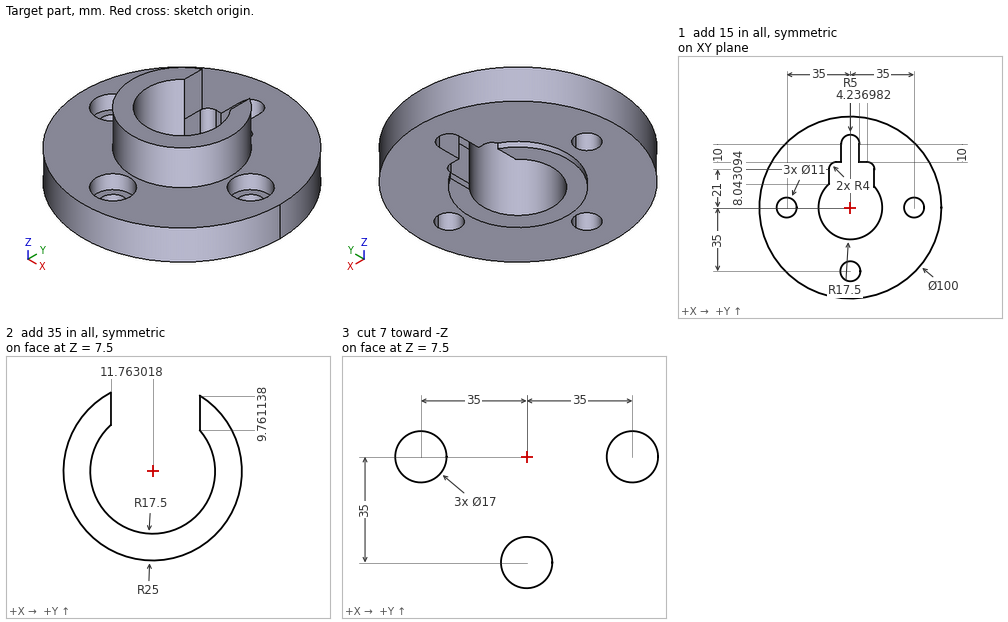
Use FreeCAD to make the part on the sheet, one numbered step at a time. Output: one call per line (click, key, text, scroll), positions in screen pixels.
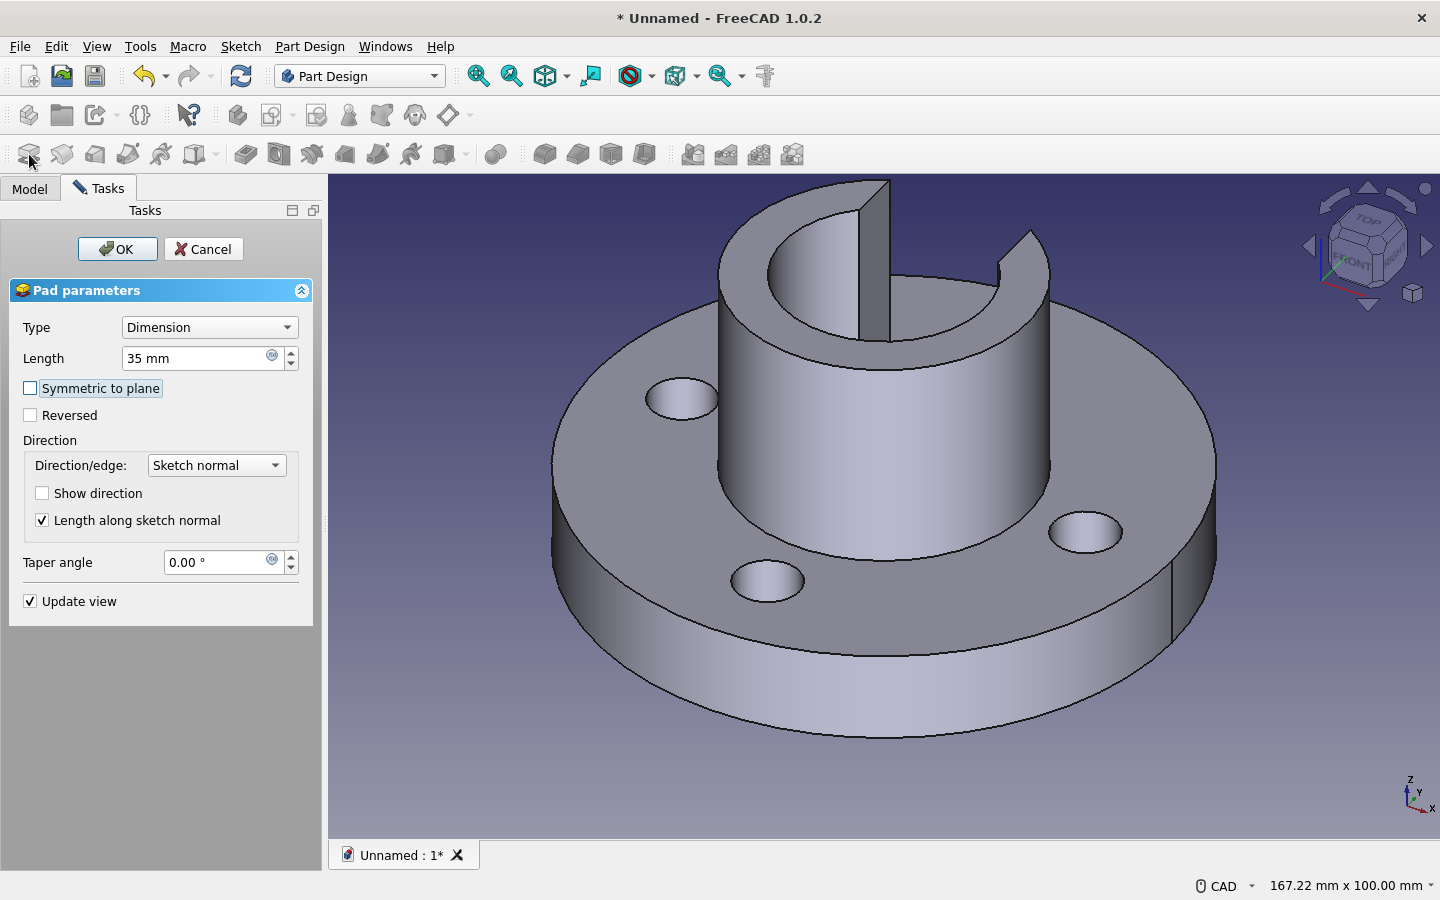
click(31, 388)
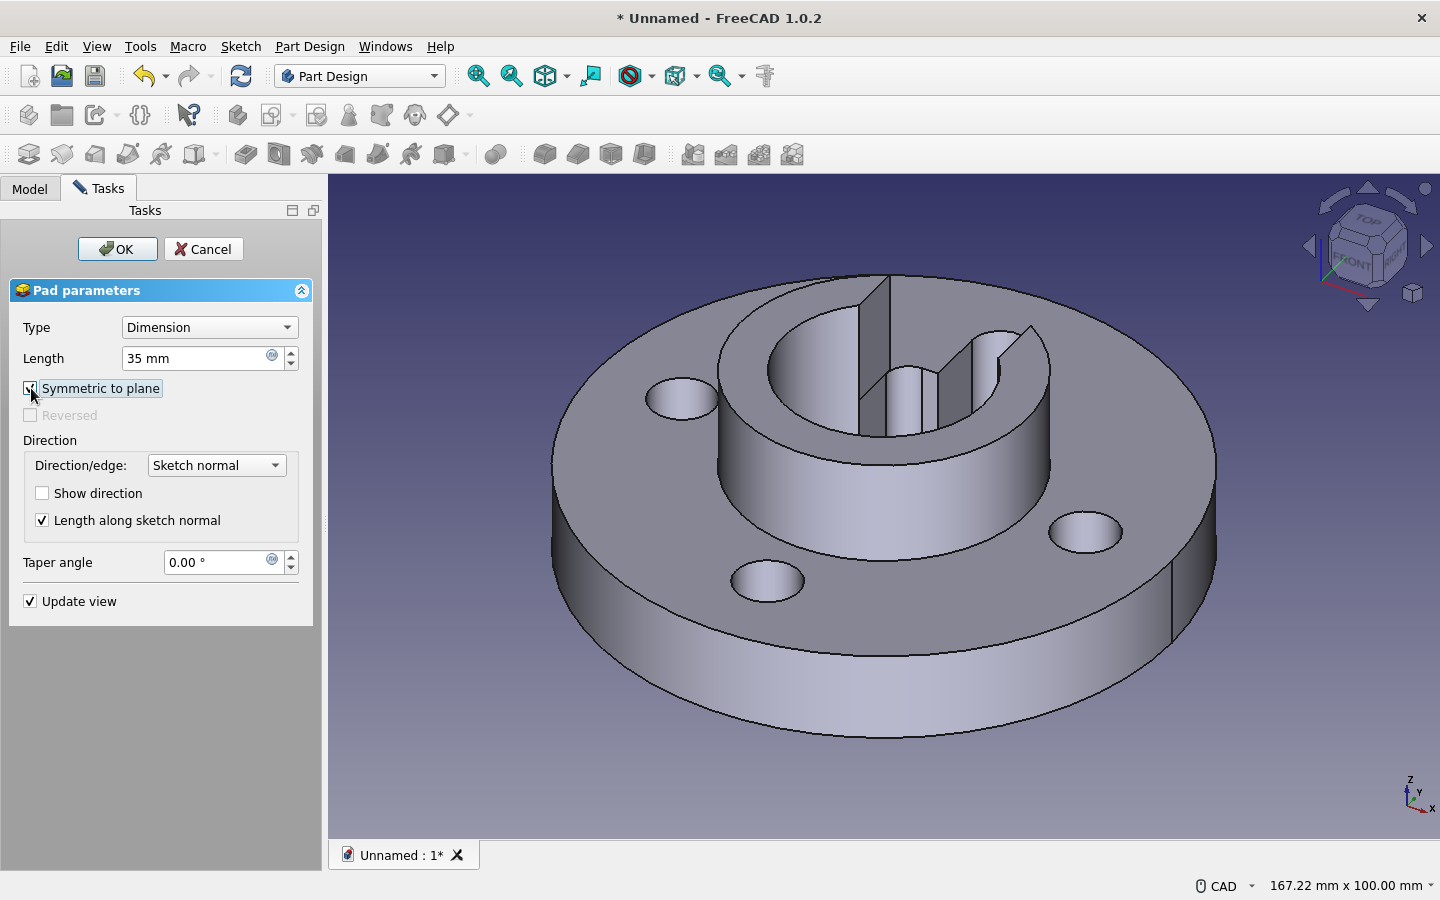
click(118, 249)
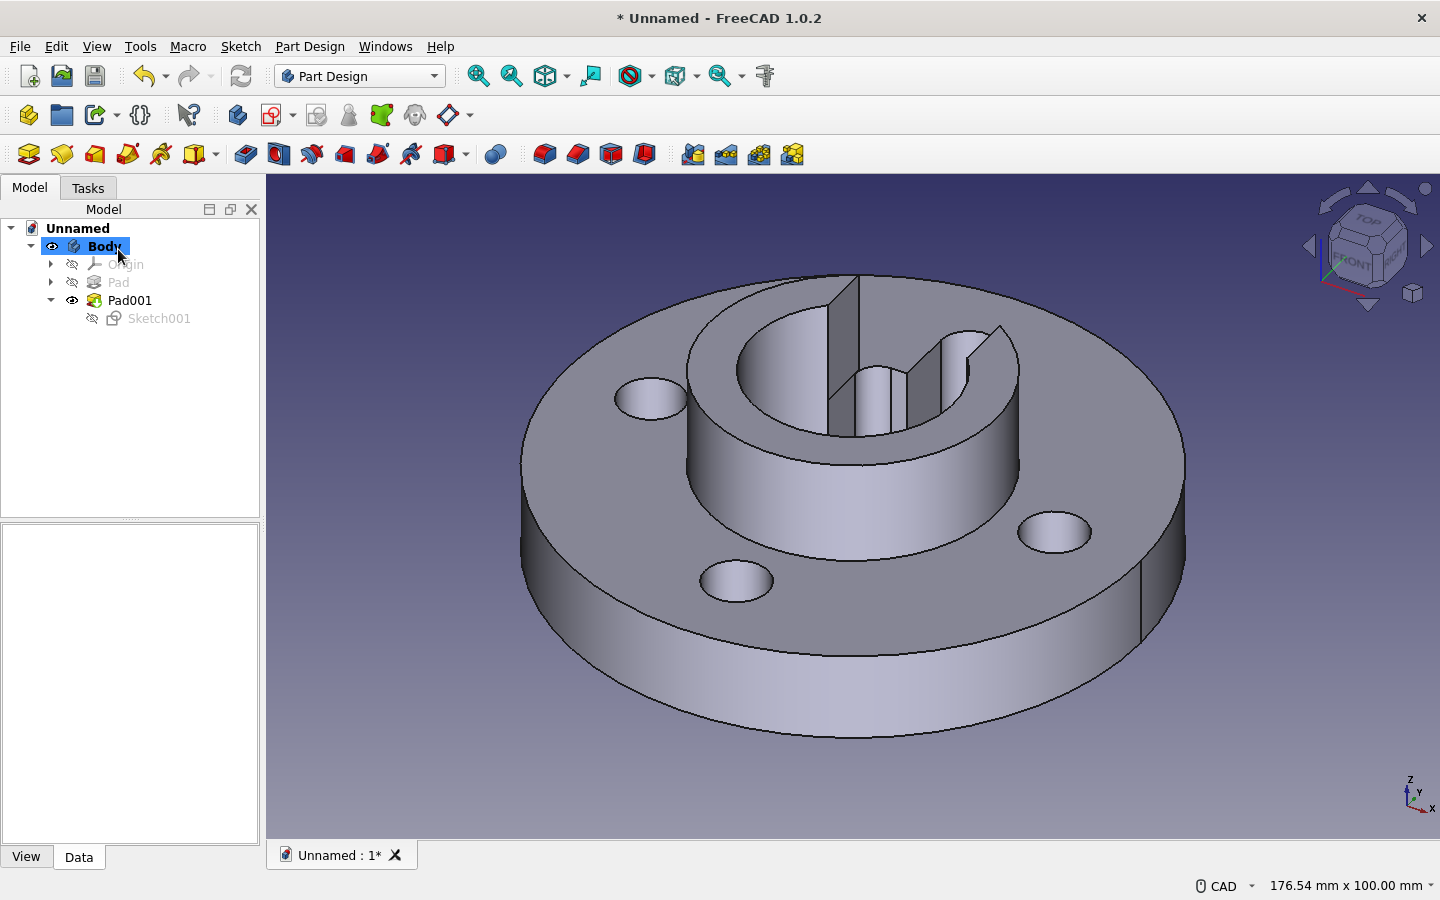
key(v)
key(f)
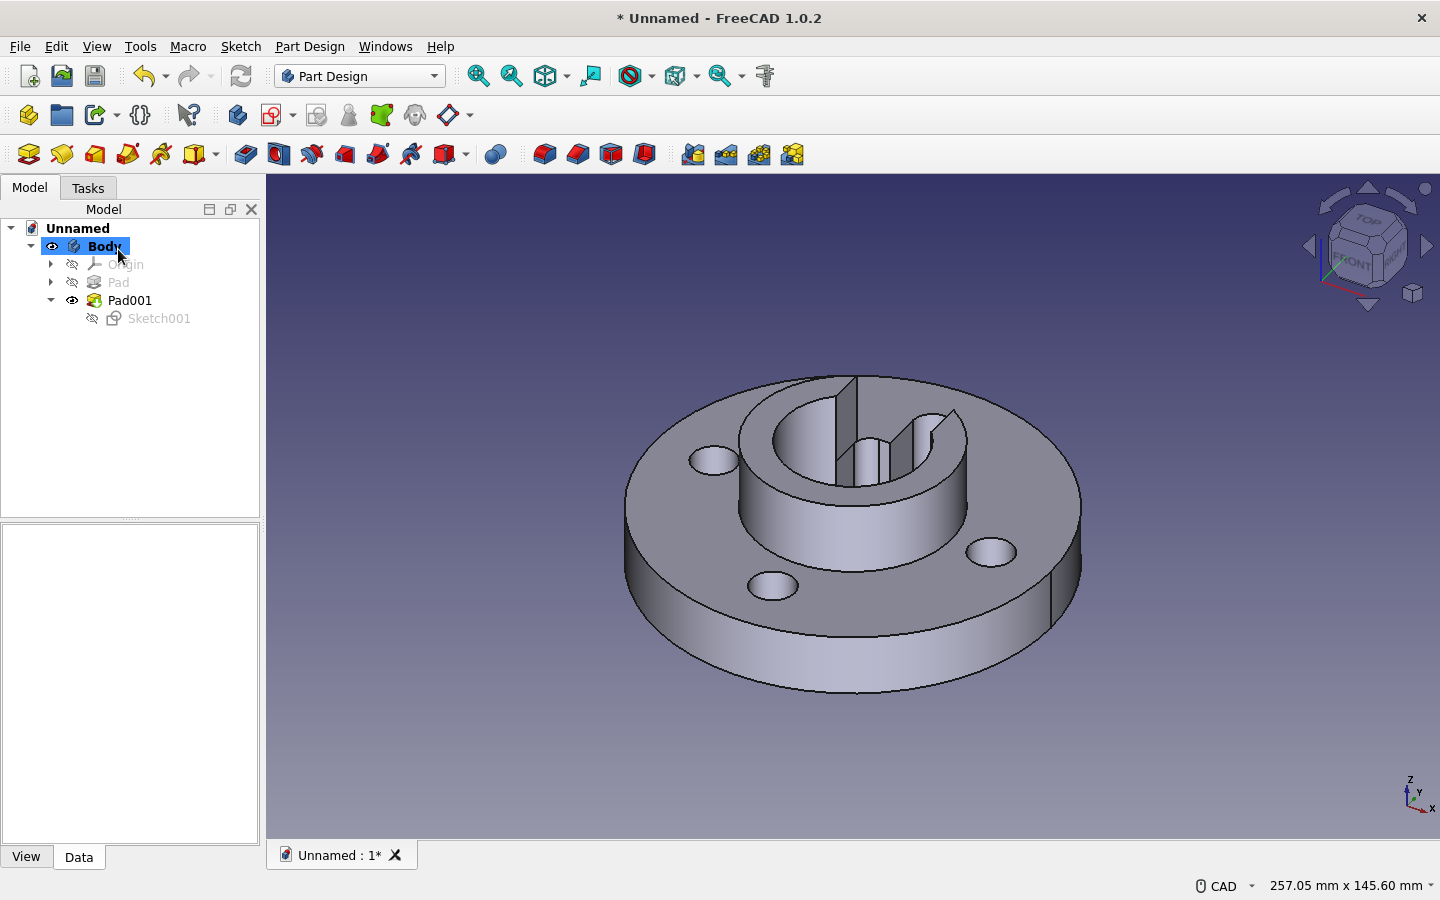
click(901, 608)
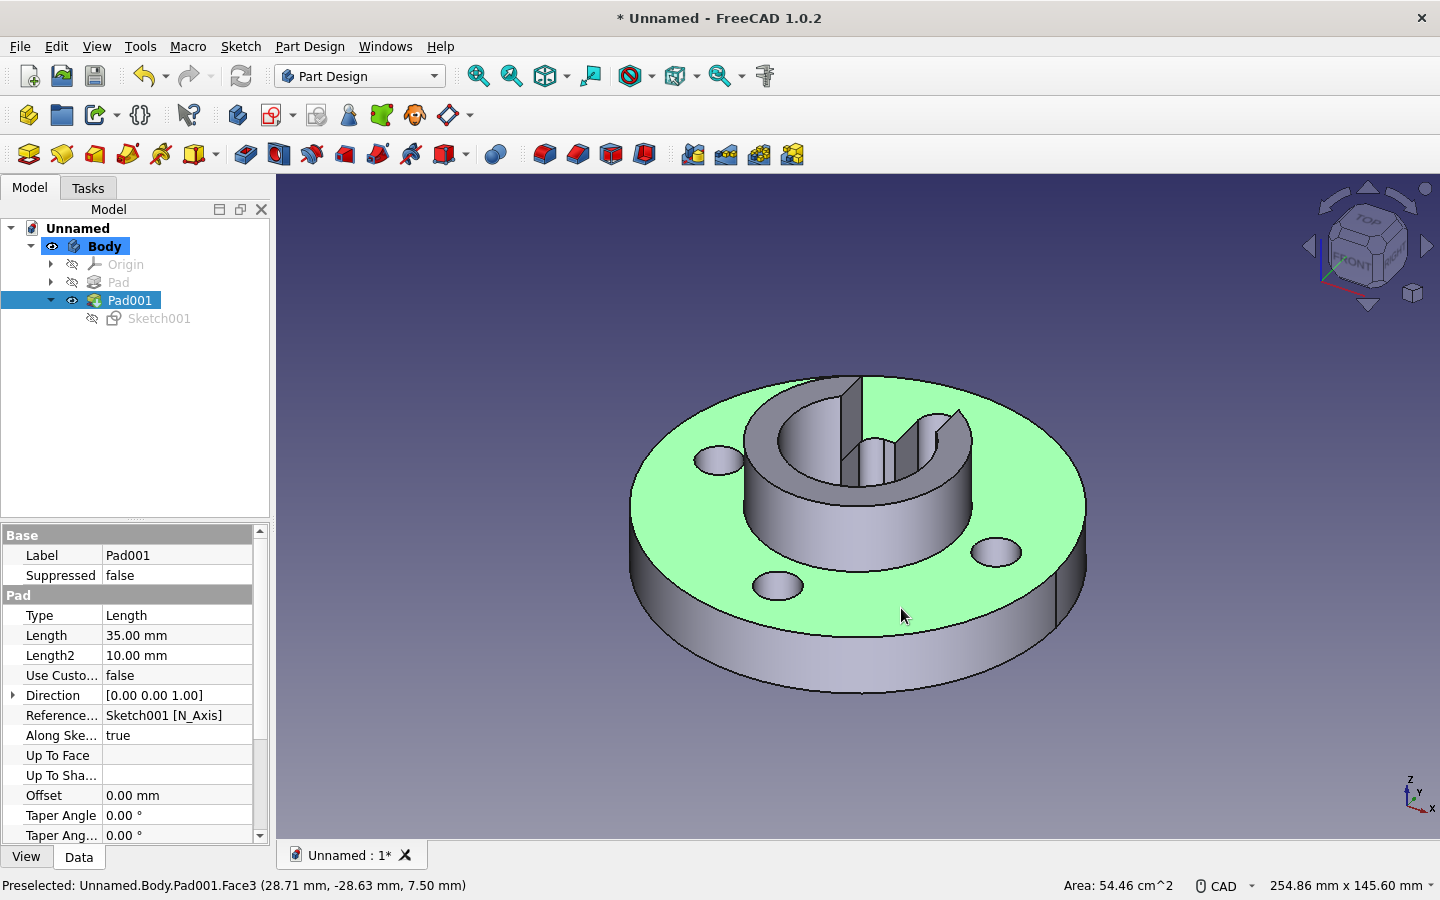
click(270, 116)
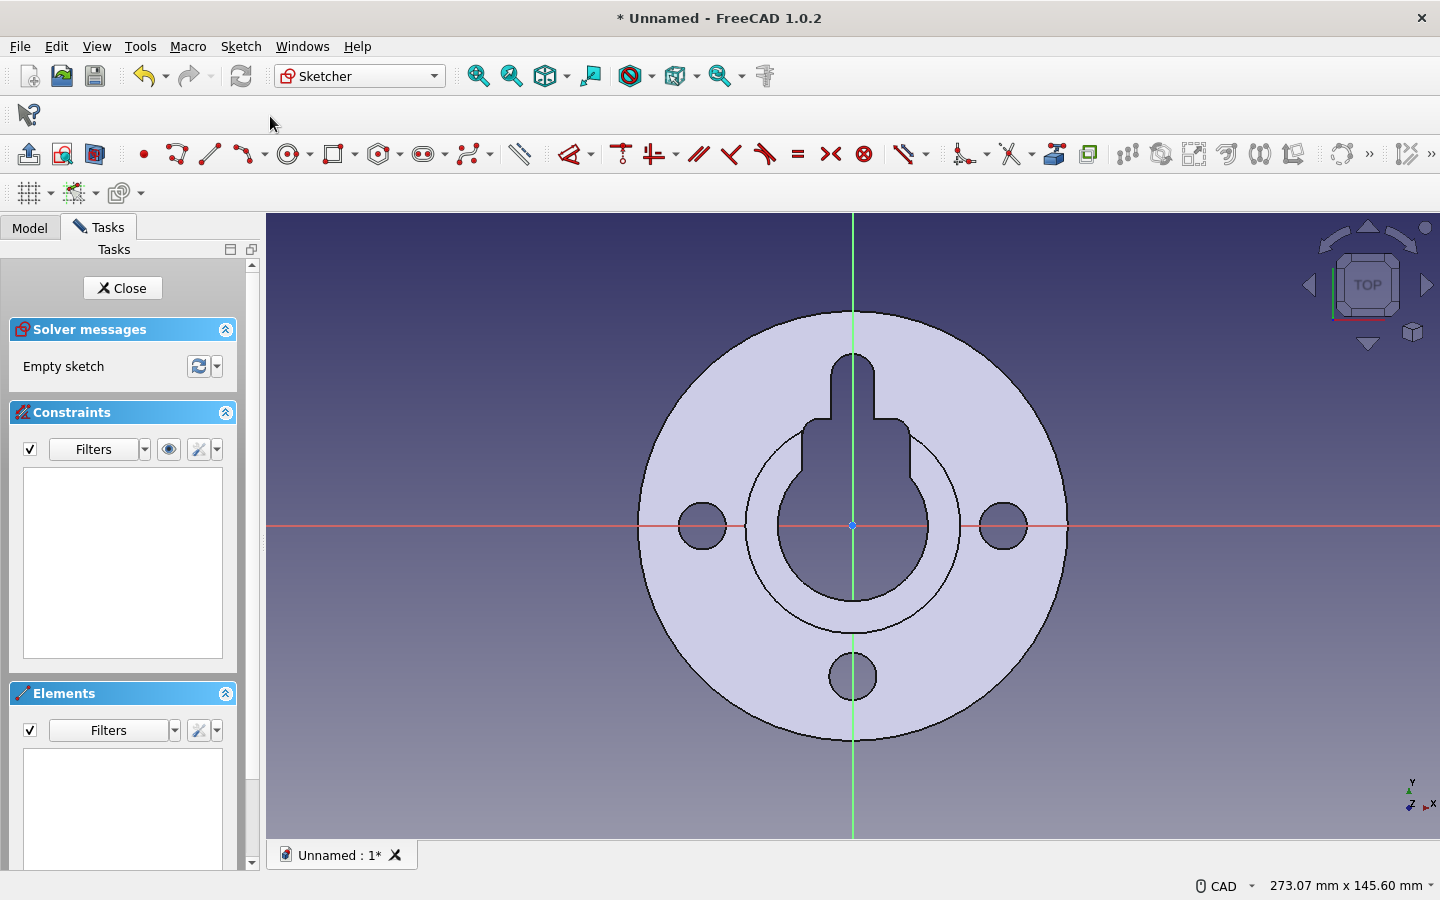
scroll(936, 693, up, 3)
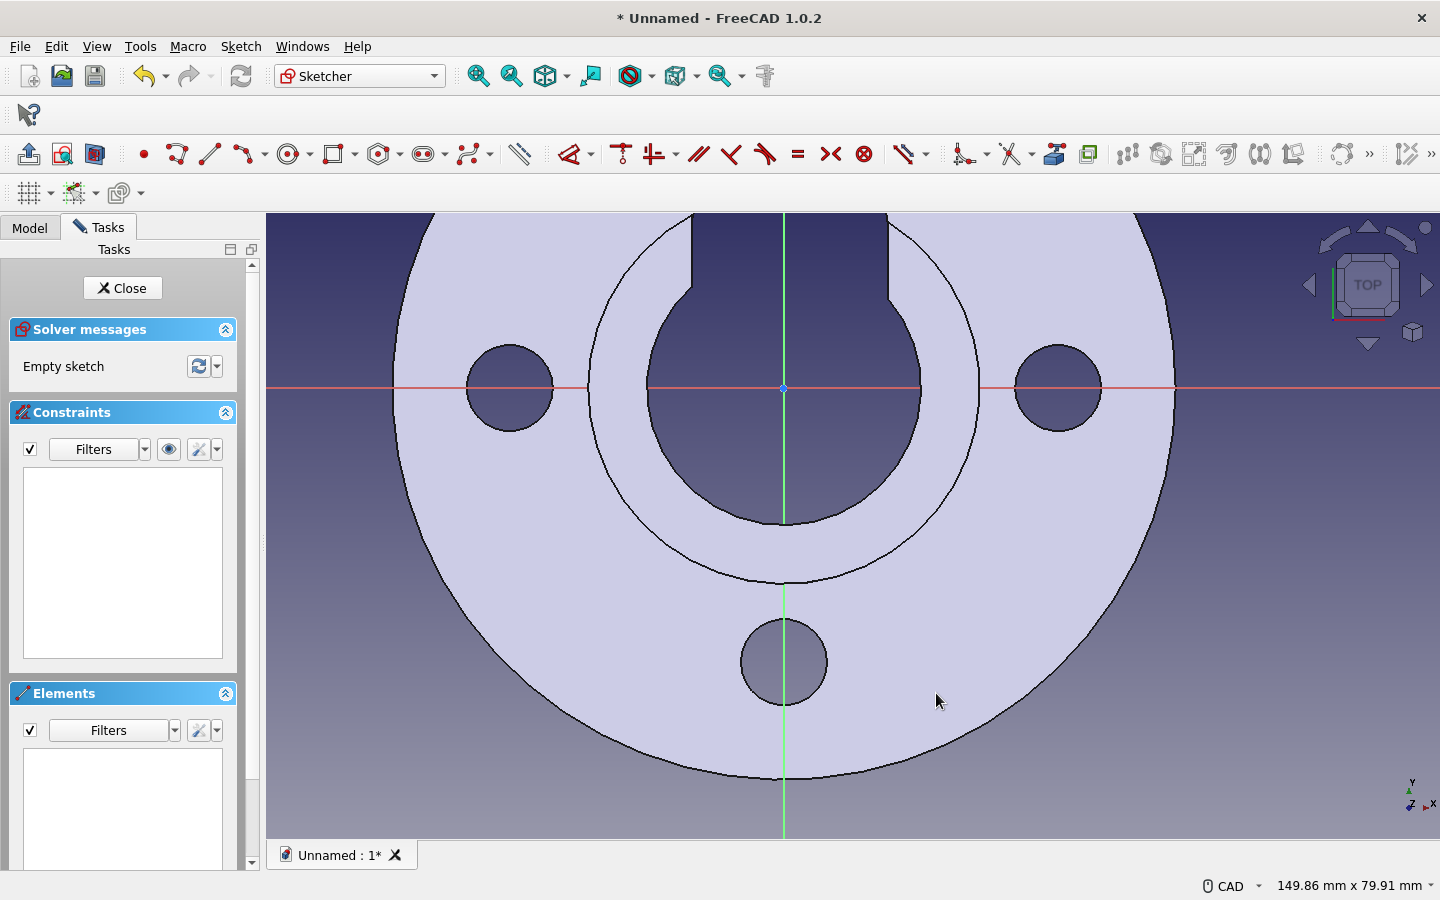
key(g)
key(c)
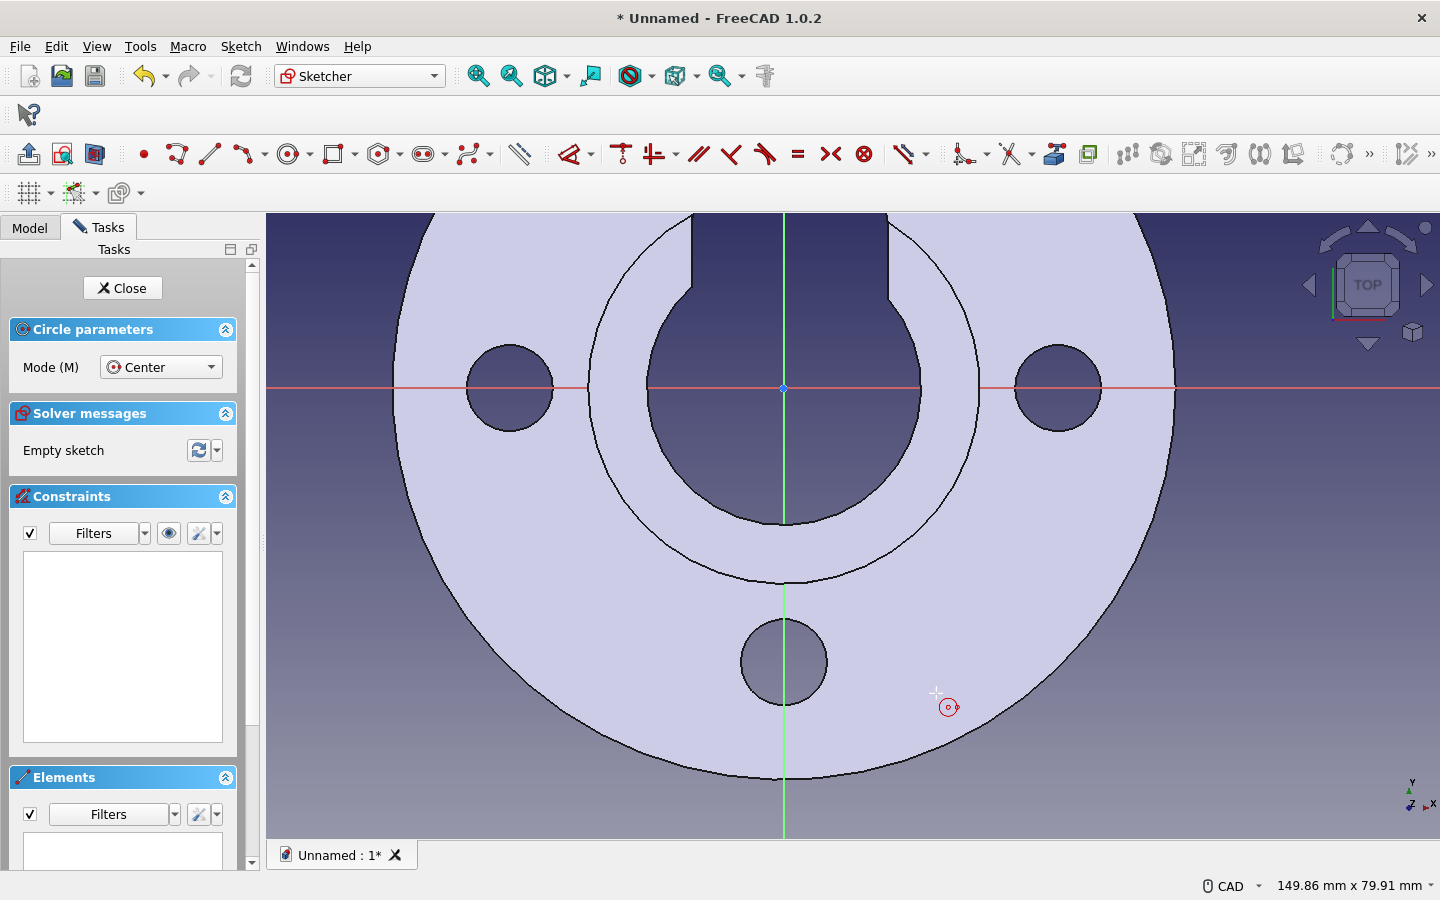
click(510, 388)
click(557, 341)